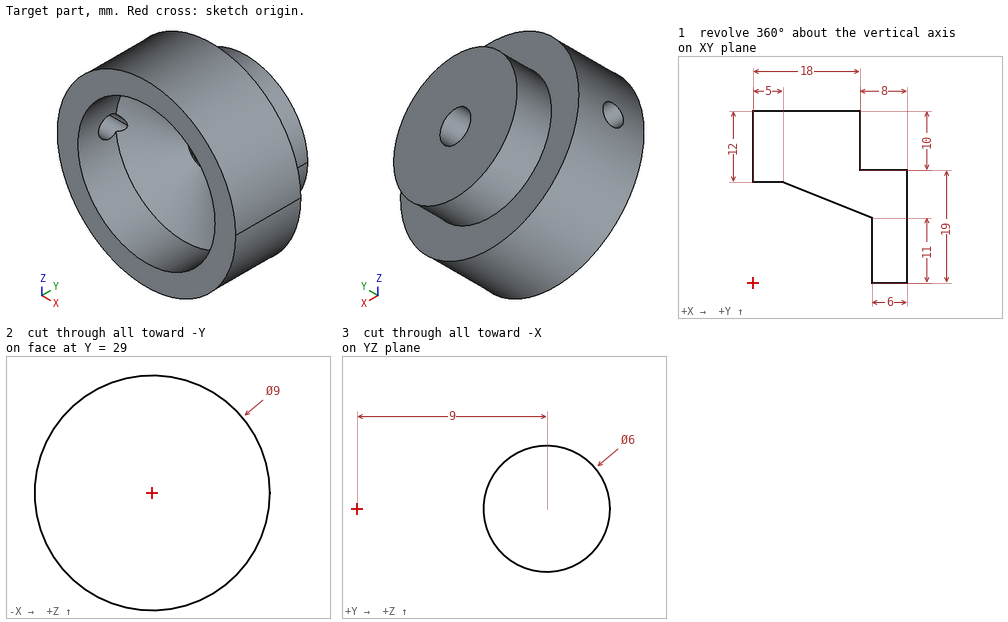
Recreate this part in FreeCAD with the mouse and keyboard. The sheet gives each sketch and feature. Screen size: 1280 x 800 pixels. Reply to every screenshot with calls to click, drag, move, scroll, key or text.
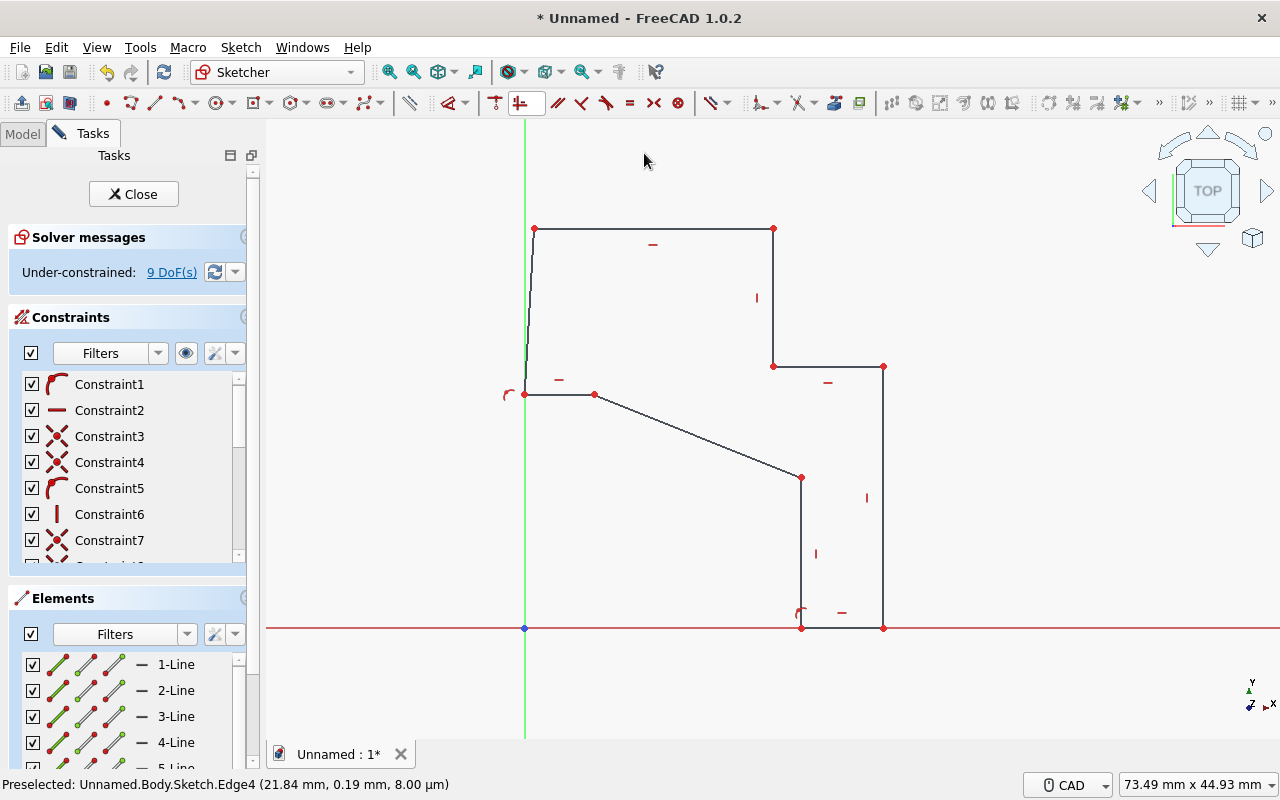
click(527, 345)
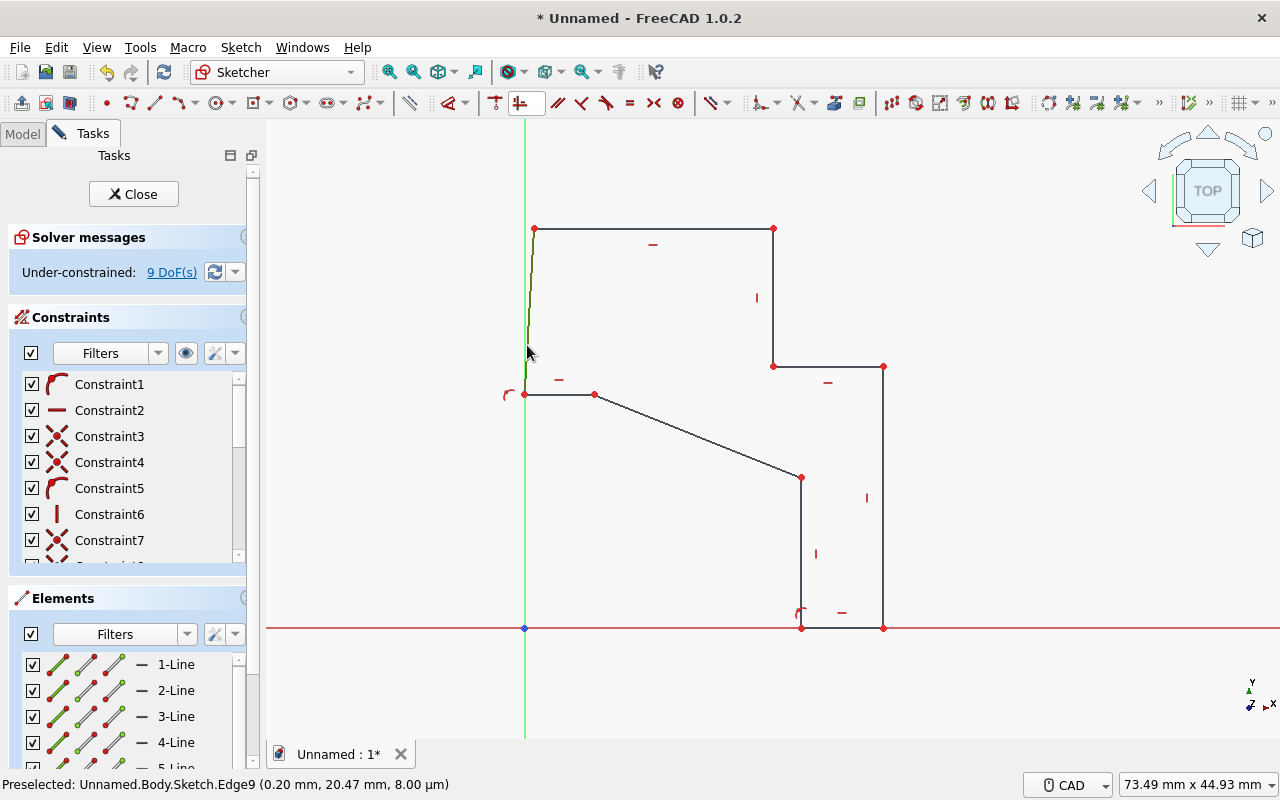
key(v)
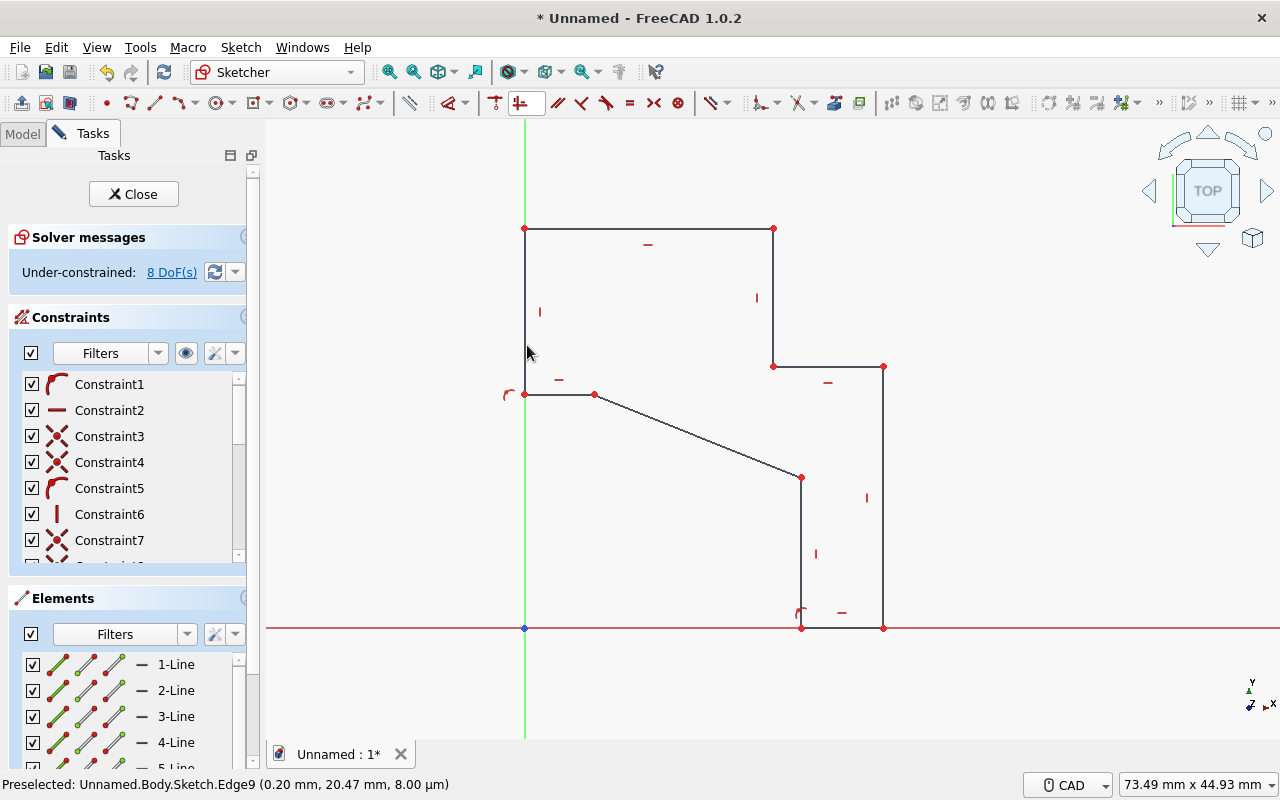
click(448, 104)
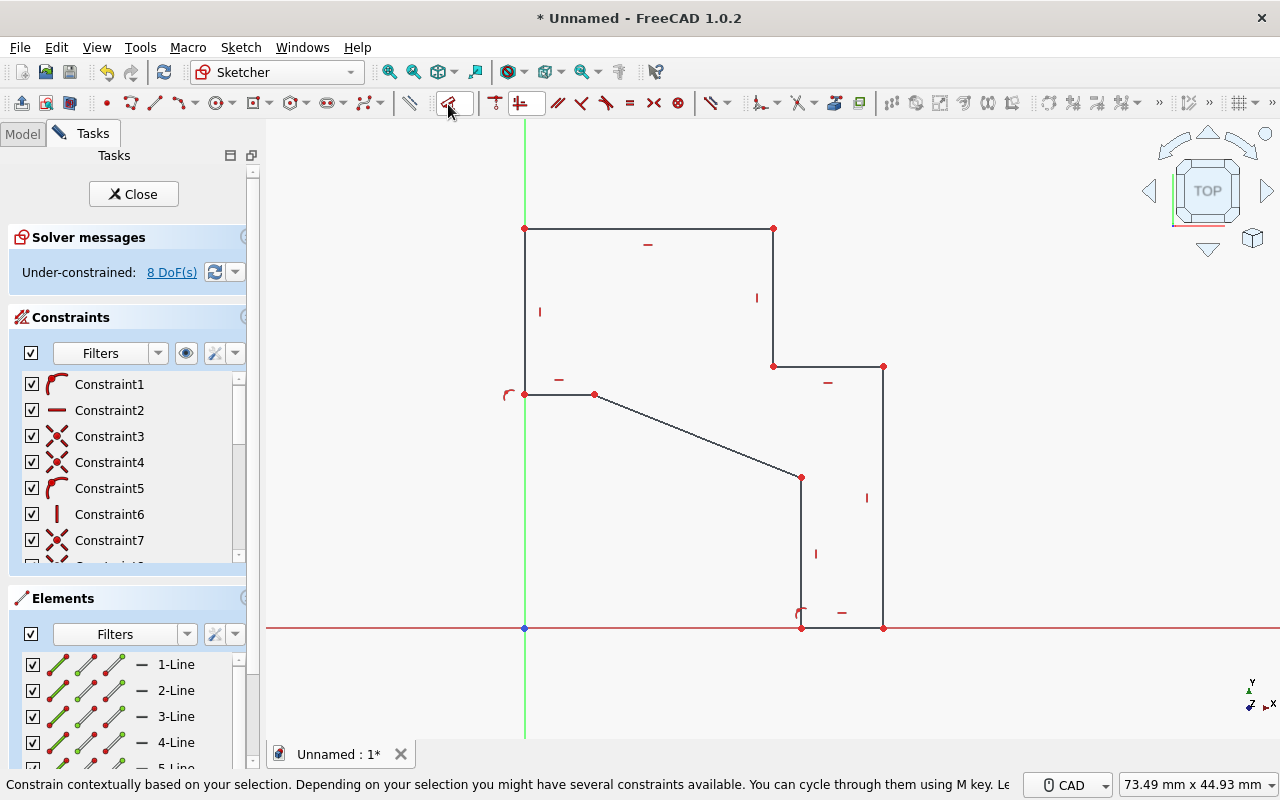
click(545, 395)
click(559, 361)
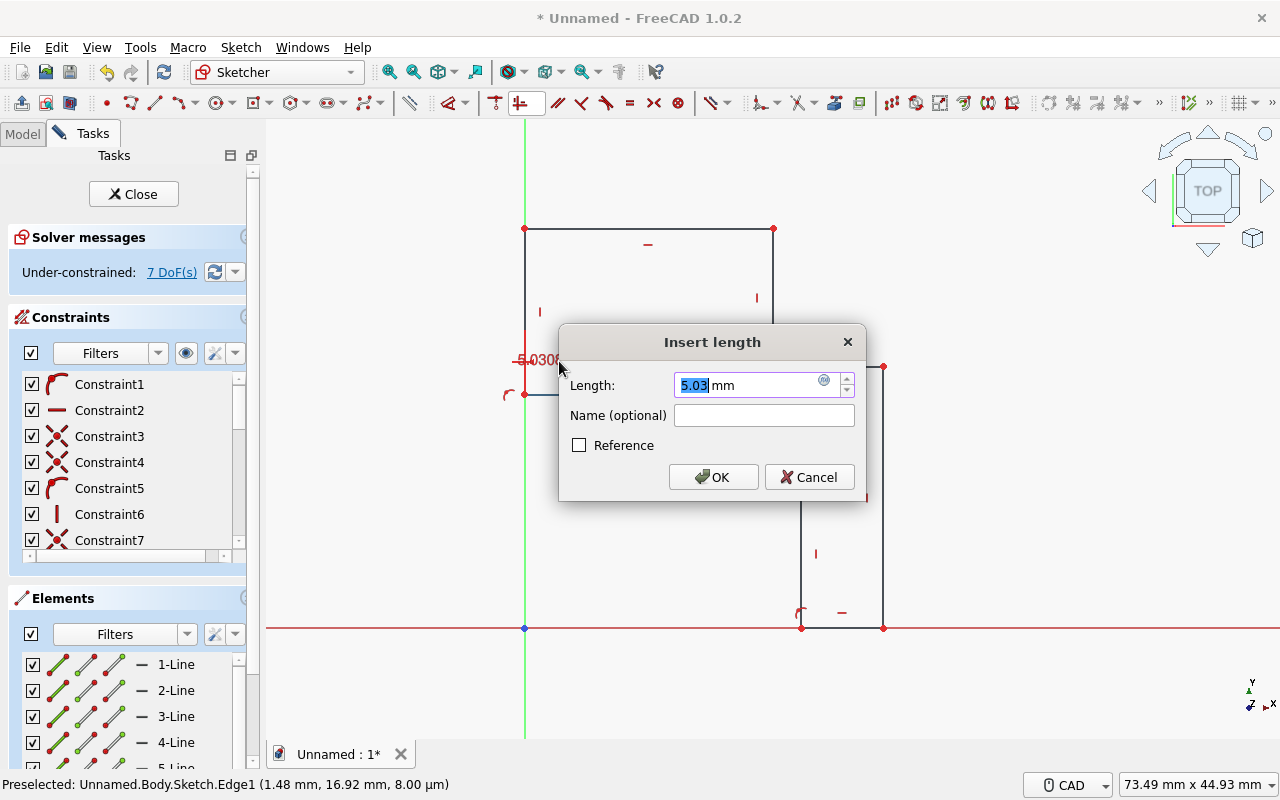
text(5)
key(Return)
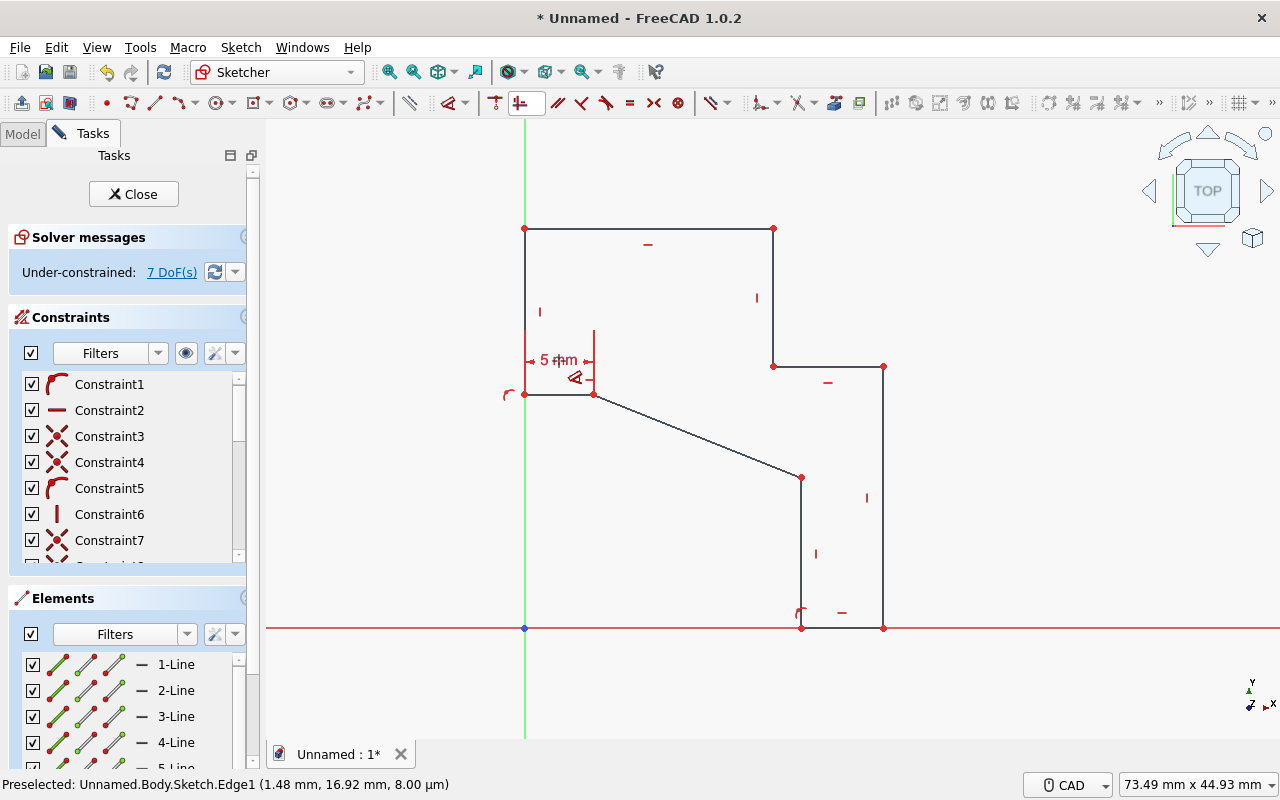
click(826, 628)
click(842, 662)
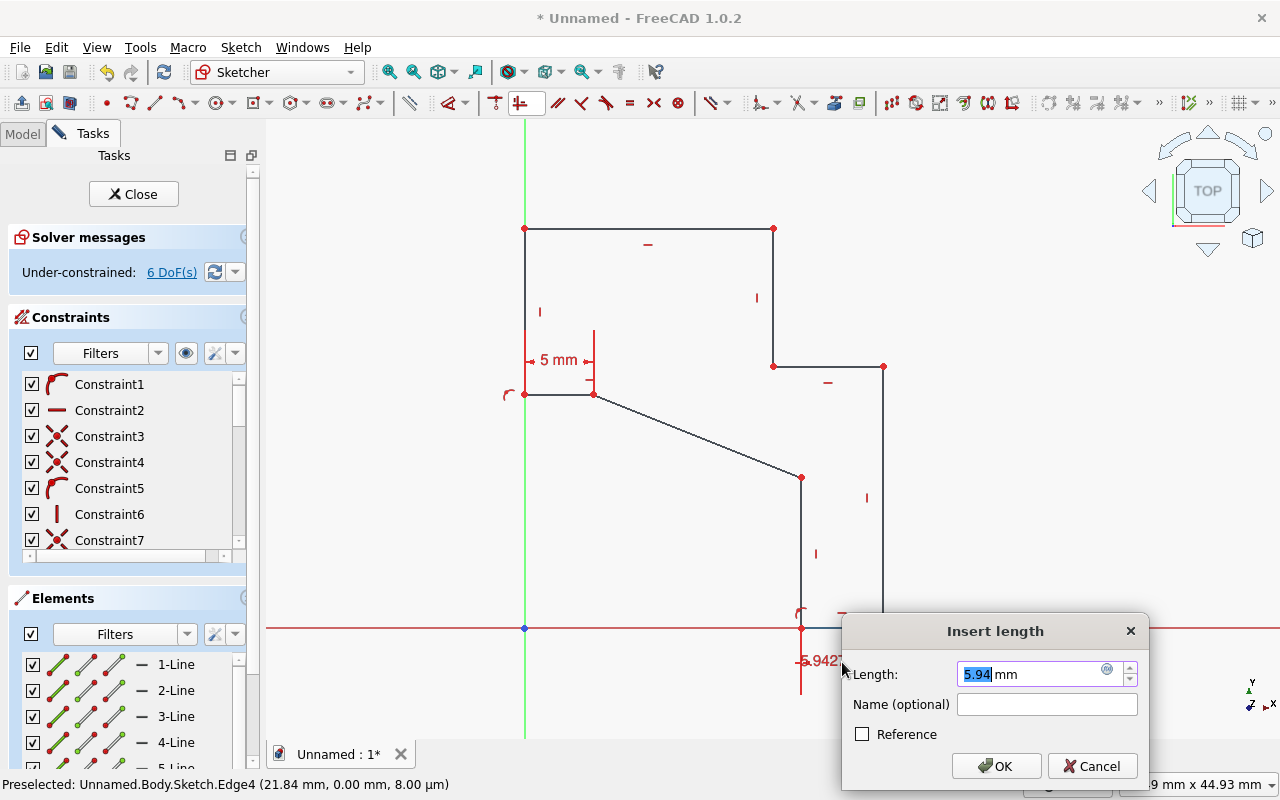
text(6)
key(Return)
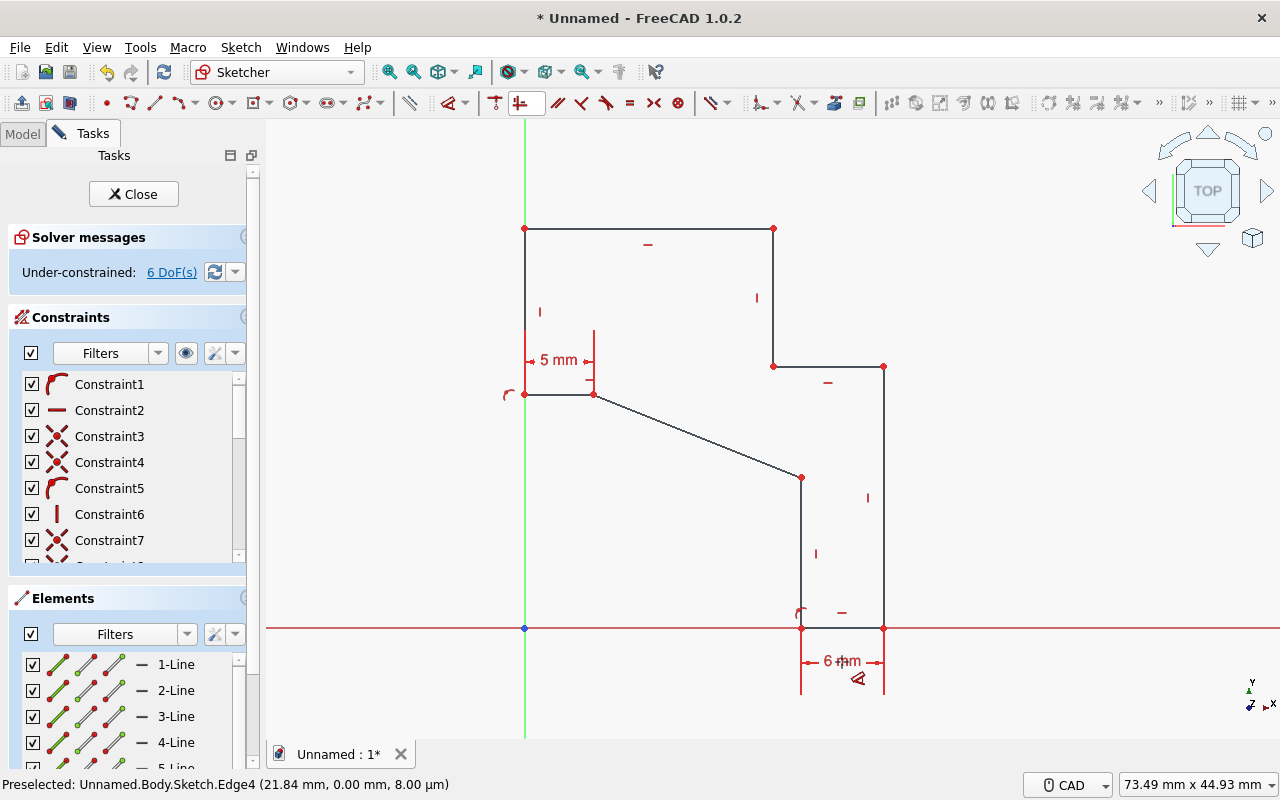
click(851, 367)
click(828, 333)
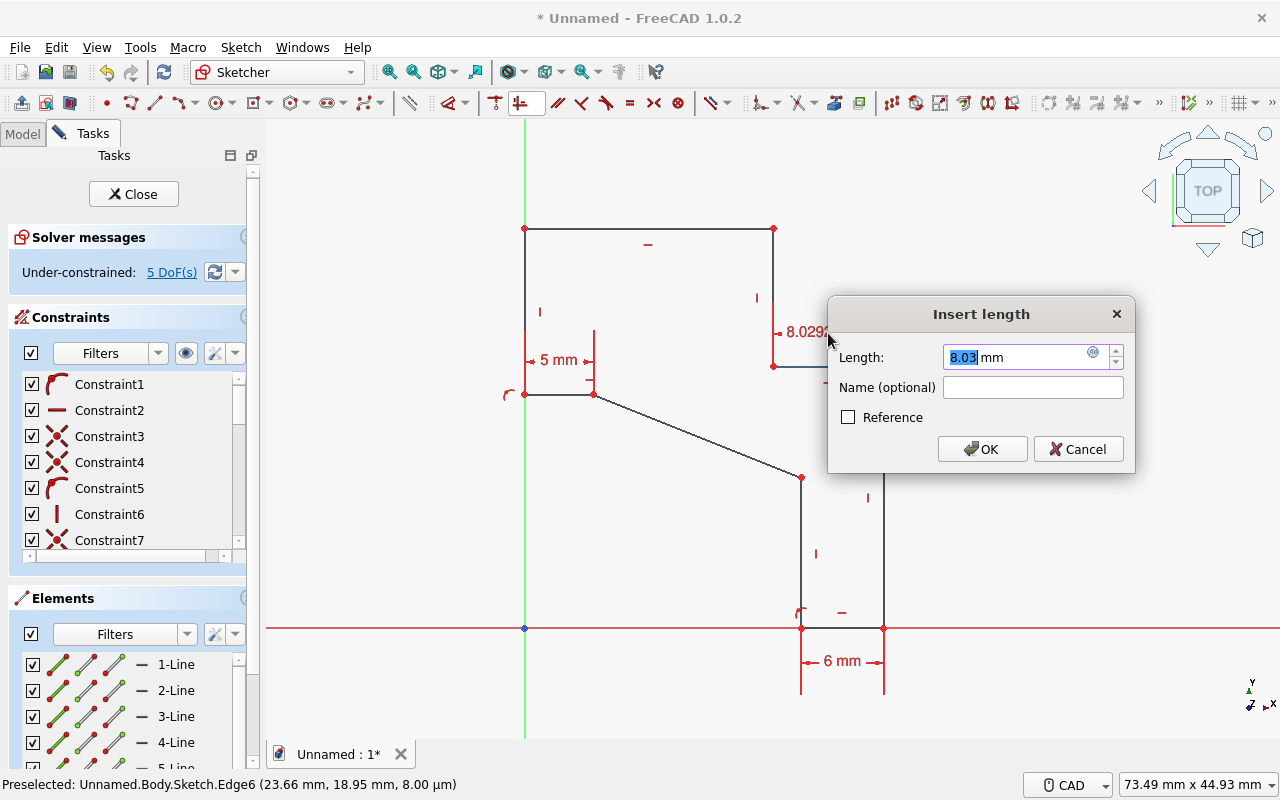
text(8)
key(Return)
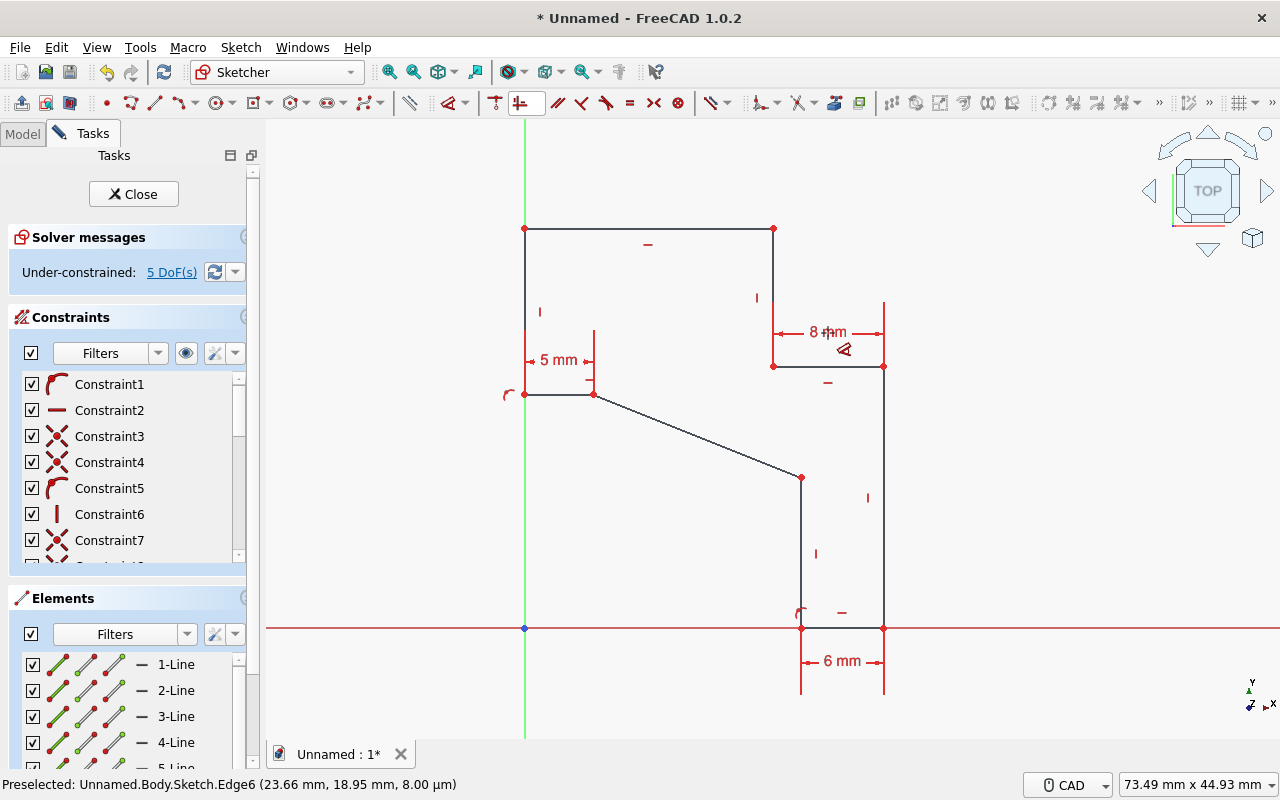
click(801, 523)
click(835, 553)